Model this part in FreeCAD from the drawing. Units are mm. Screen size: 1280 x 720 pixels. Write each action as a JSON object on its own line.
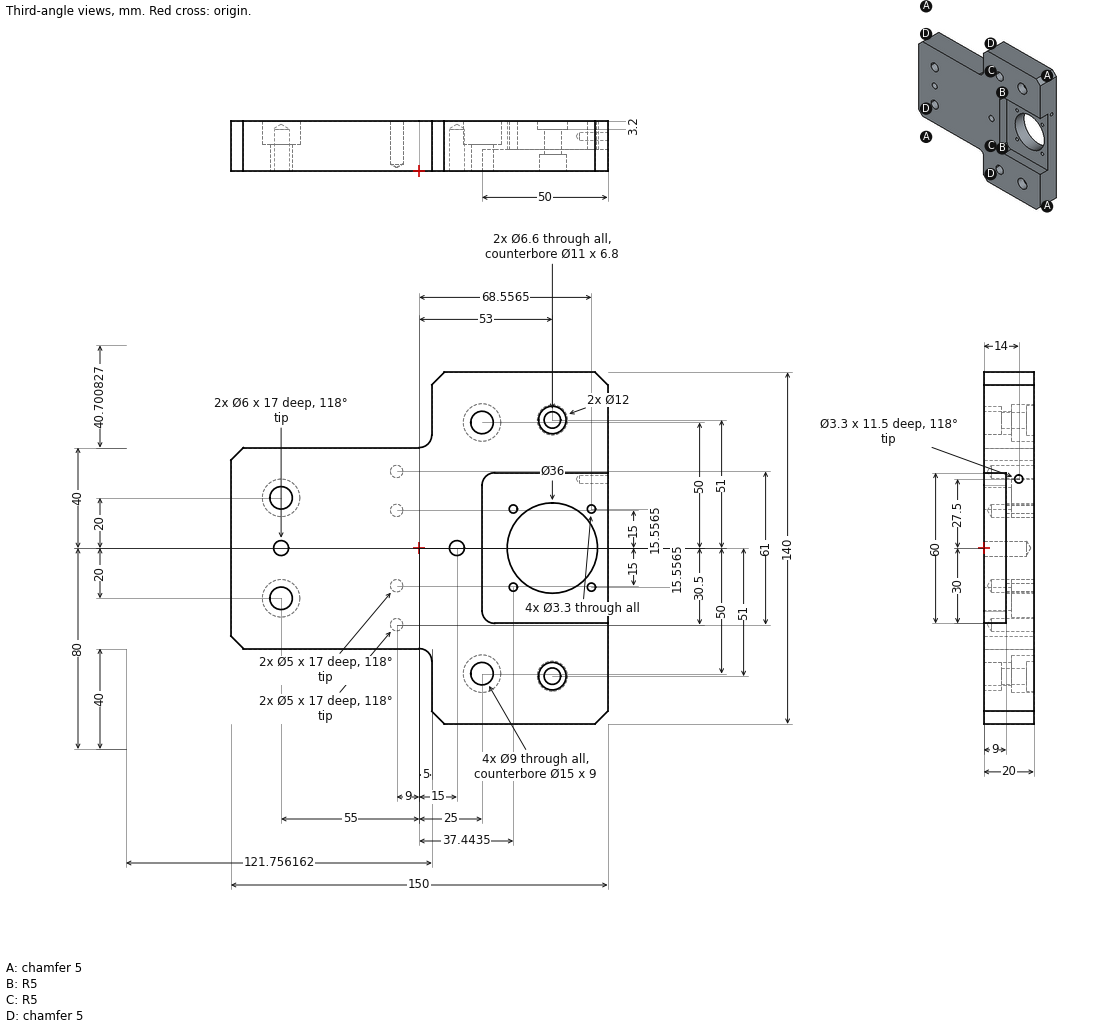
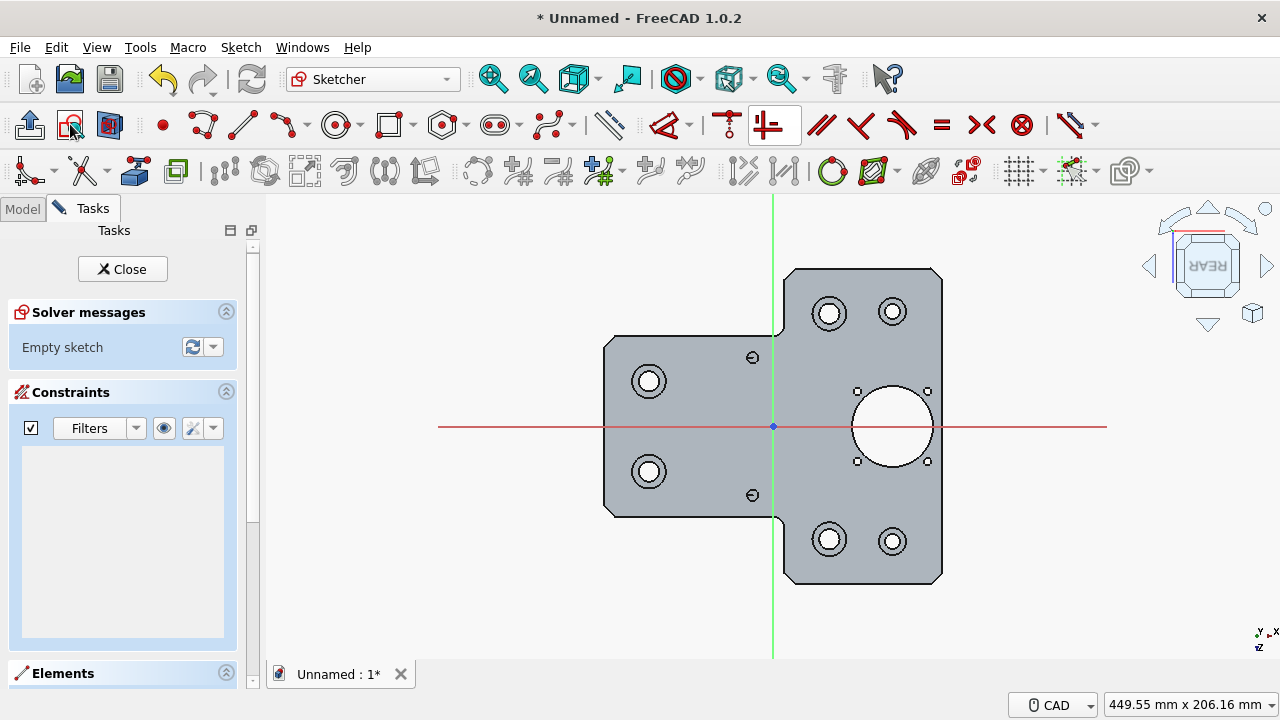
{"action": "scroll", "coordinate": [784, 426], "scroll_direction": "up", "scroll_amount": 6}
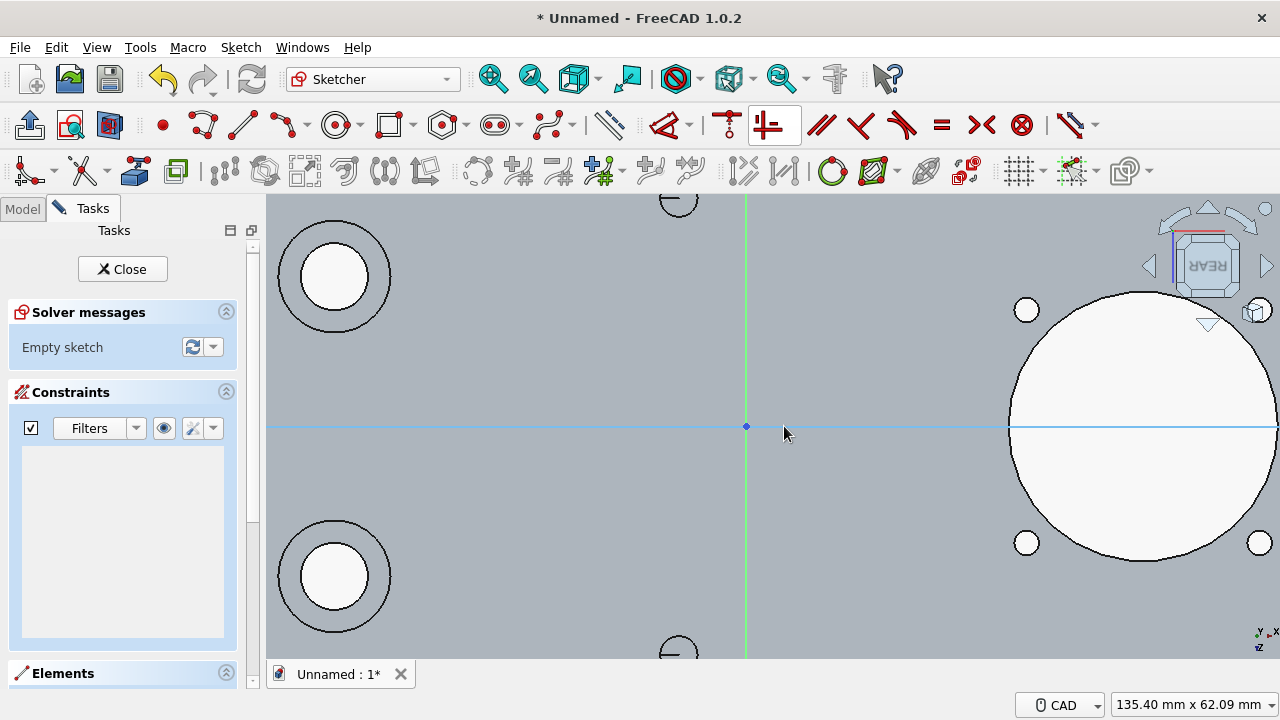
{"action": "left_click", "coordinate": [336, 126]}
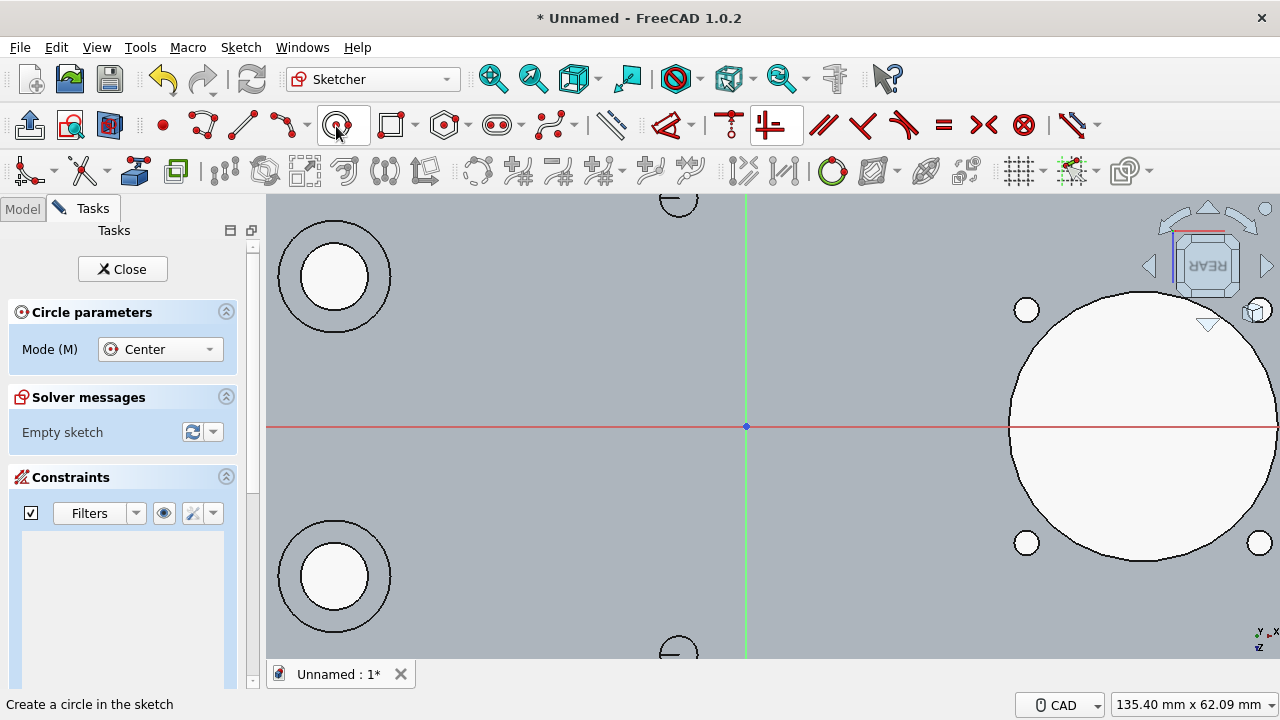
{"action": "left_click", "coordinate": [679, 314]}
{"action": "left_click", "coordinate": [692, 301]}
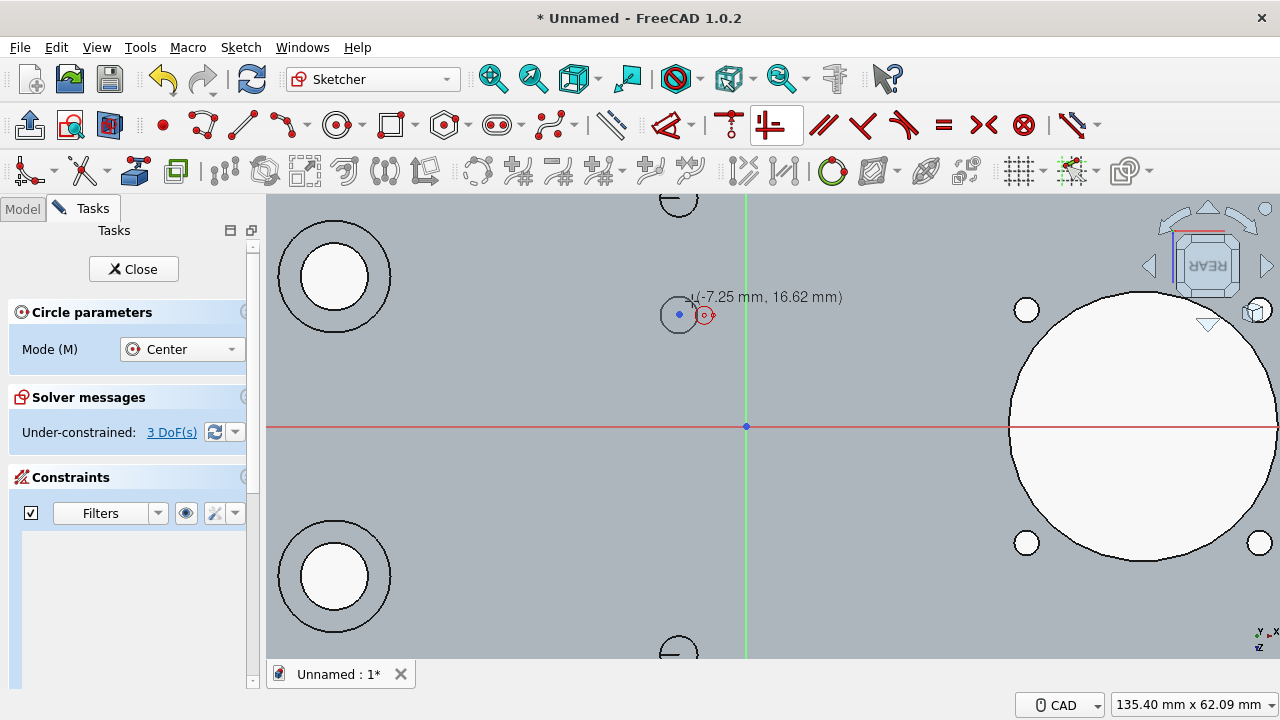
{"action": "left_click", "coordinate": [679, 539]}
{"action": "left_click", "coordinate": [692, 526]}
{"action": "key", "text": "Escape"}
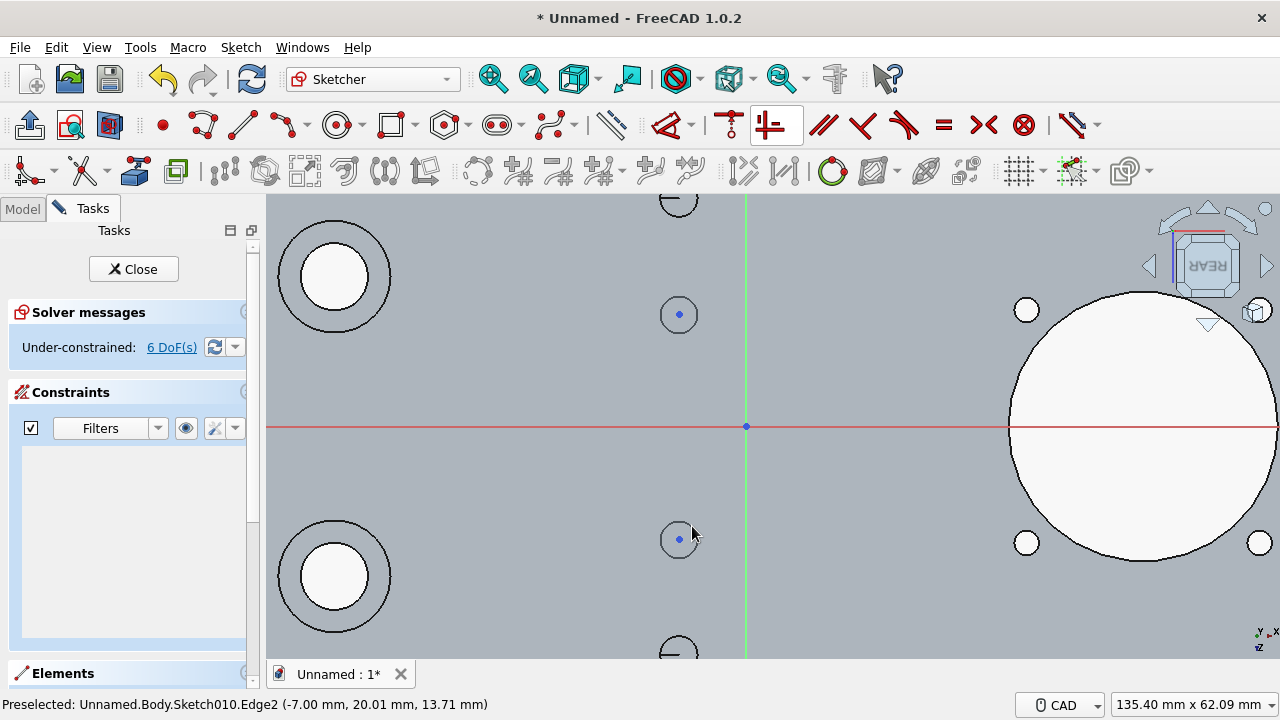
{"action": "left_click", "coordinate": [692, 302]}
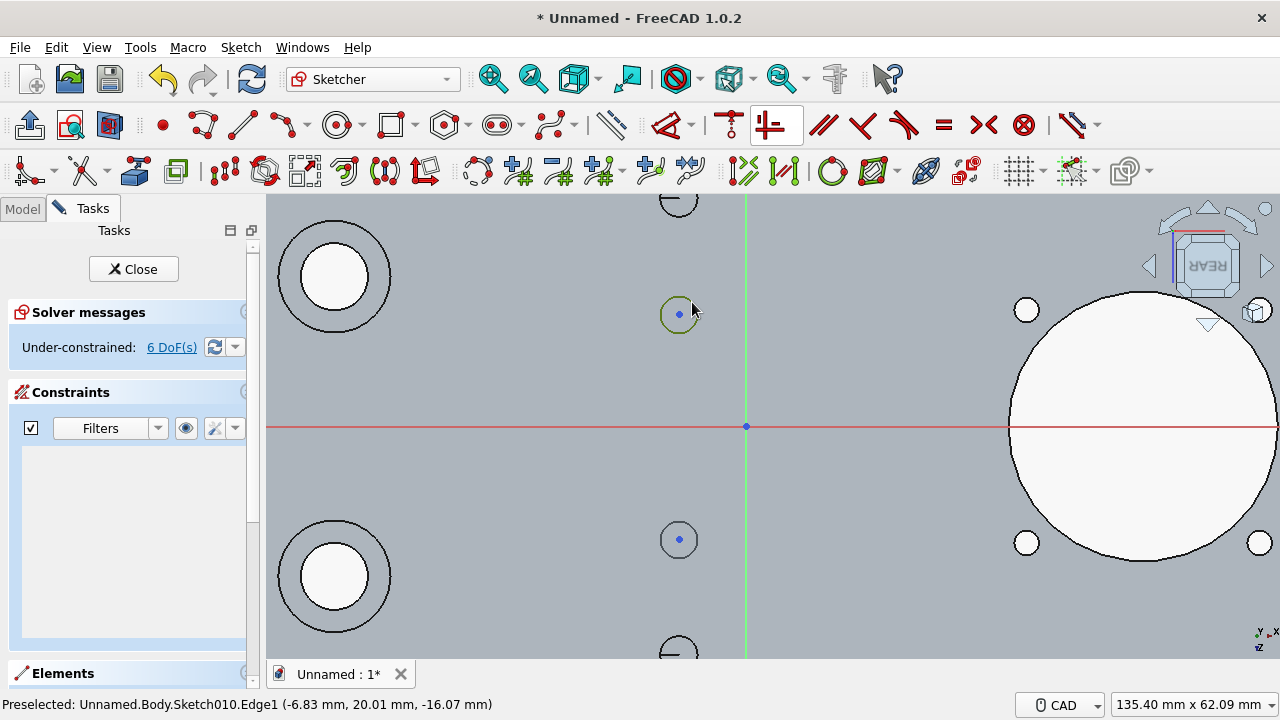
{"action": "left_click", "coordinate": [692, 527]}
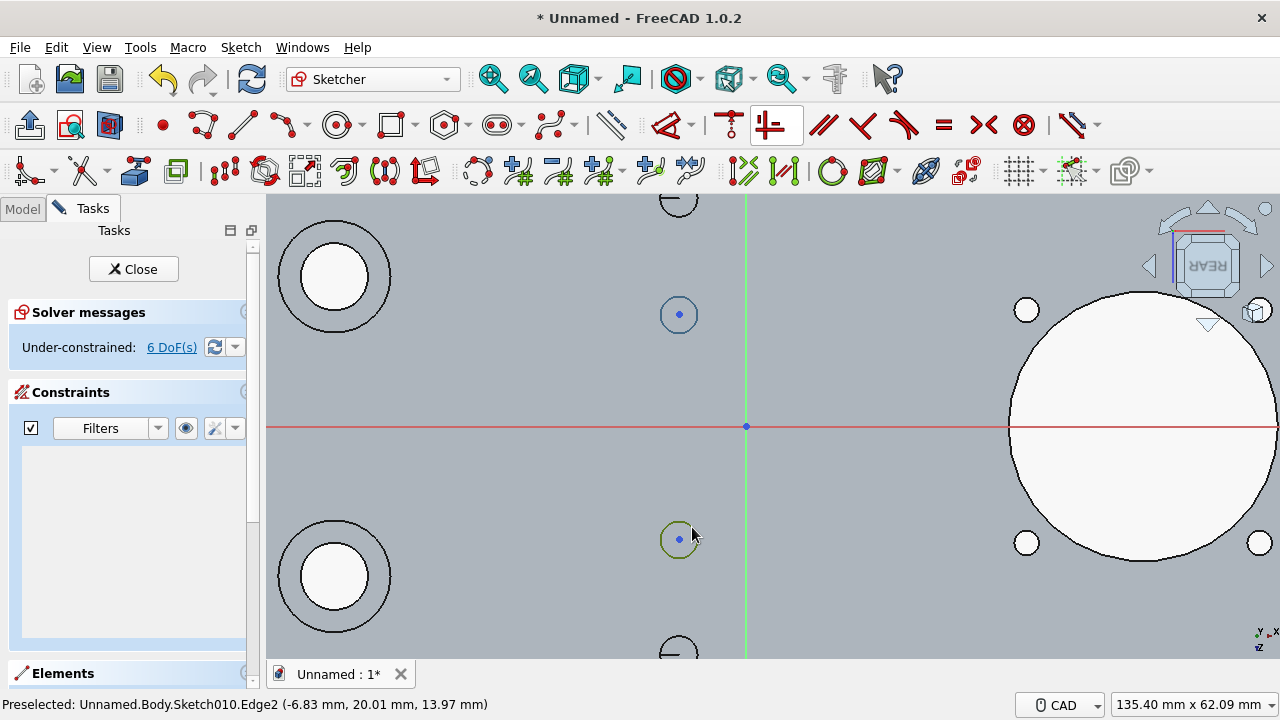
{"action": "left_click", "coordinate": [944, 126]}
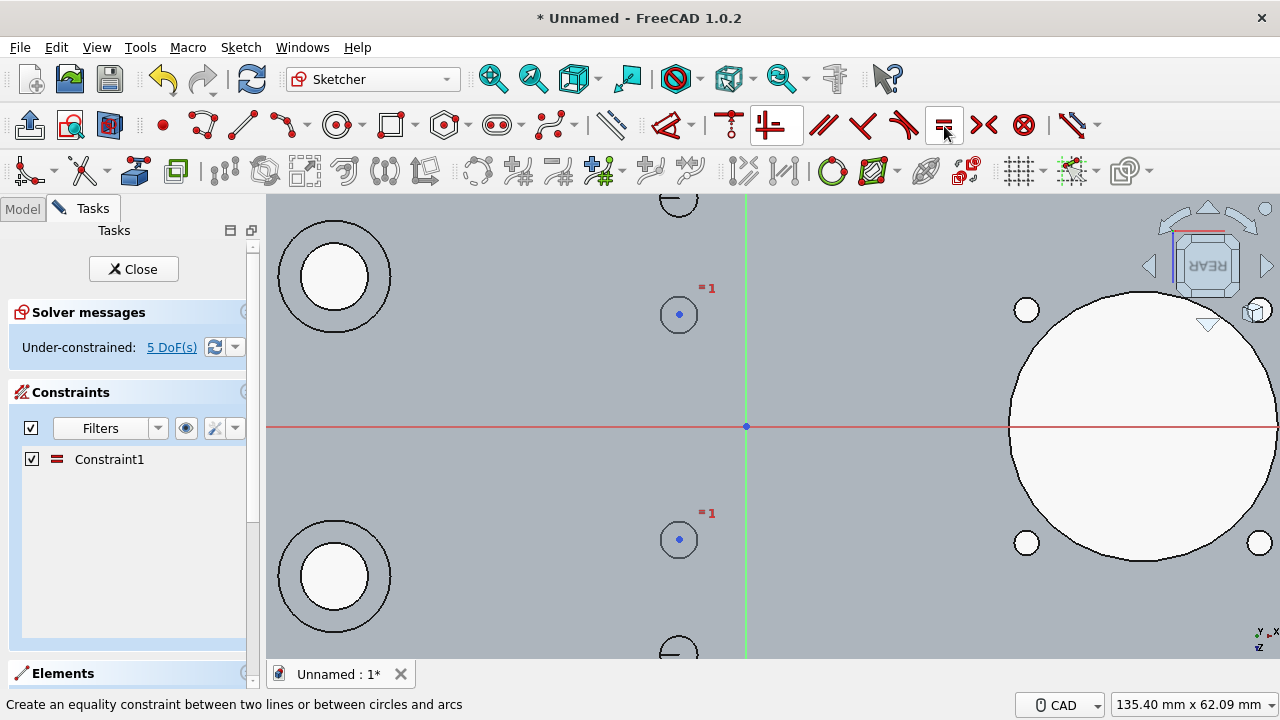
{"action": "left_click", "coordinate": [679, 315]}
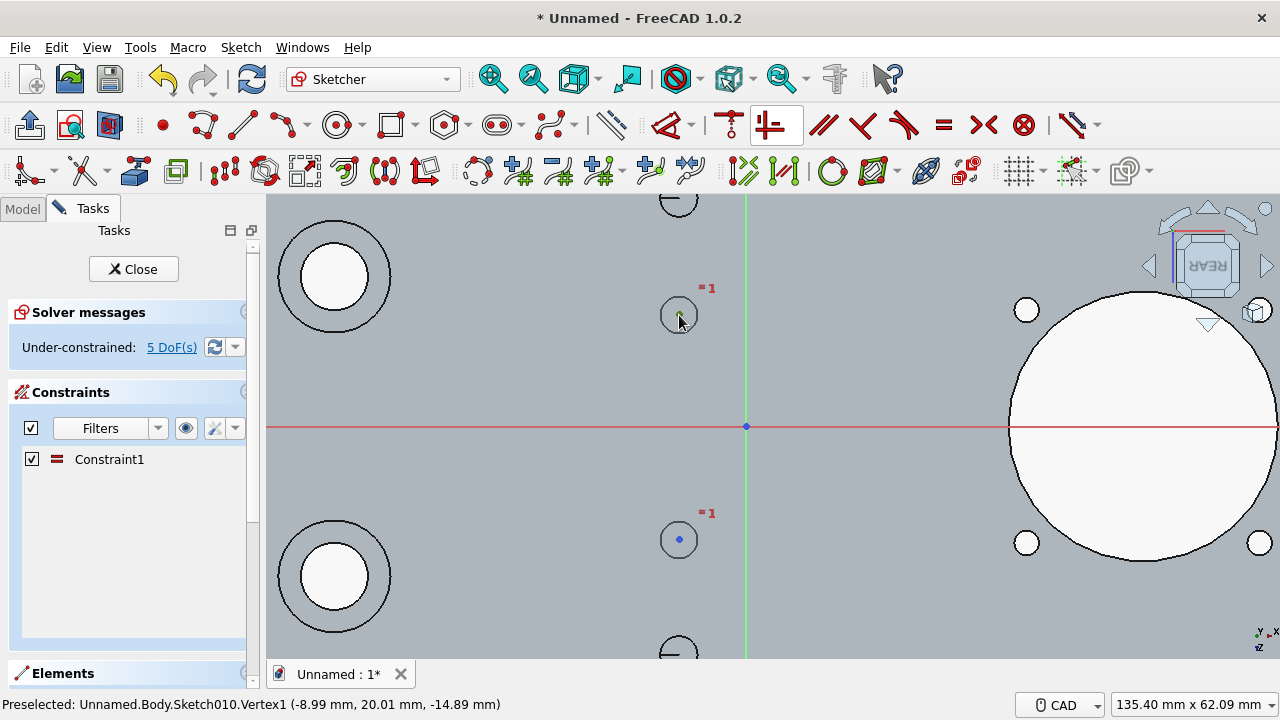
{"action": "left_click", "coordinate": [679, 540]}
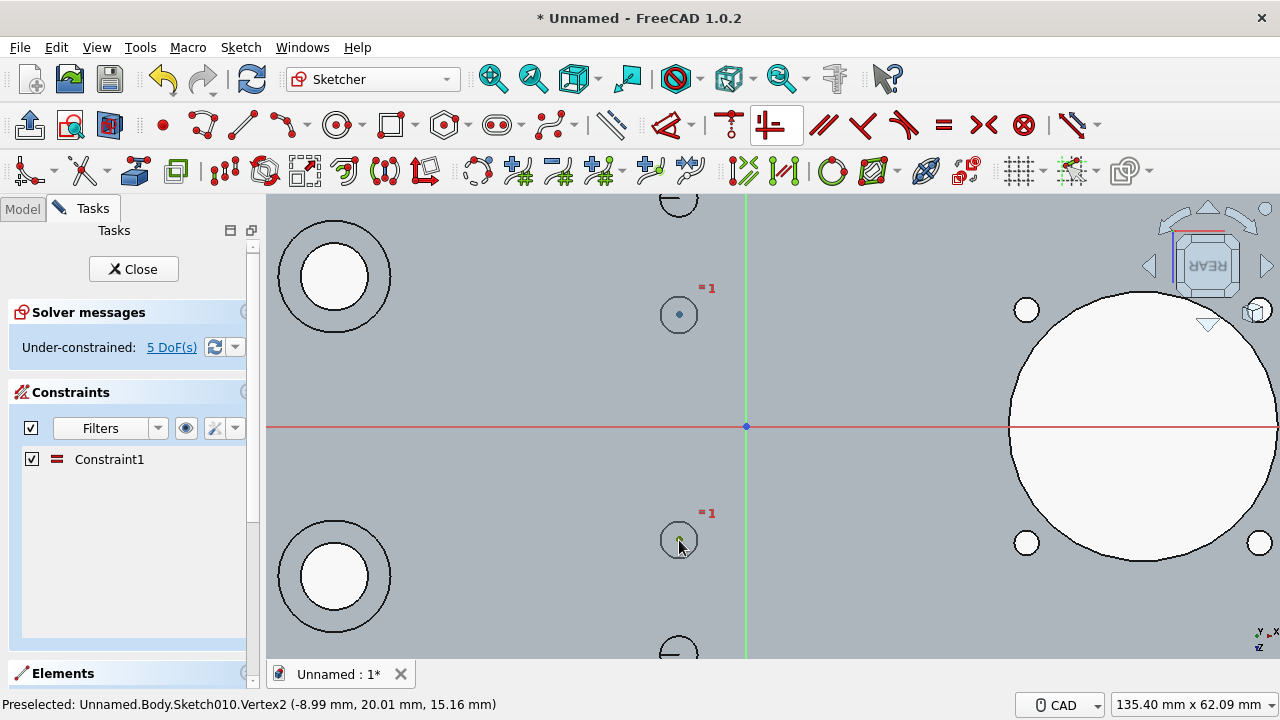
{"action": "left_click", "coordinate": [798, 126]}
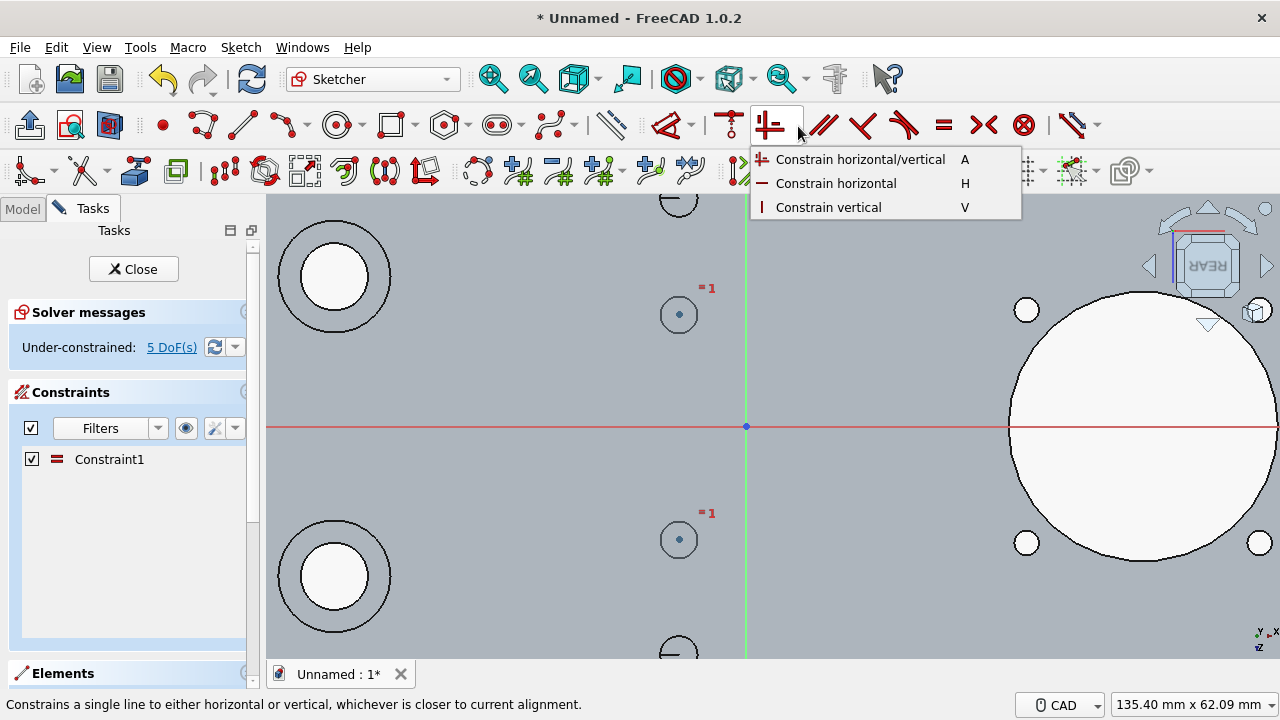
{"action": "left_click", "coordinate": [886, 207]}